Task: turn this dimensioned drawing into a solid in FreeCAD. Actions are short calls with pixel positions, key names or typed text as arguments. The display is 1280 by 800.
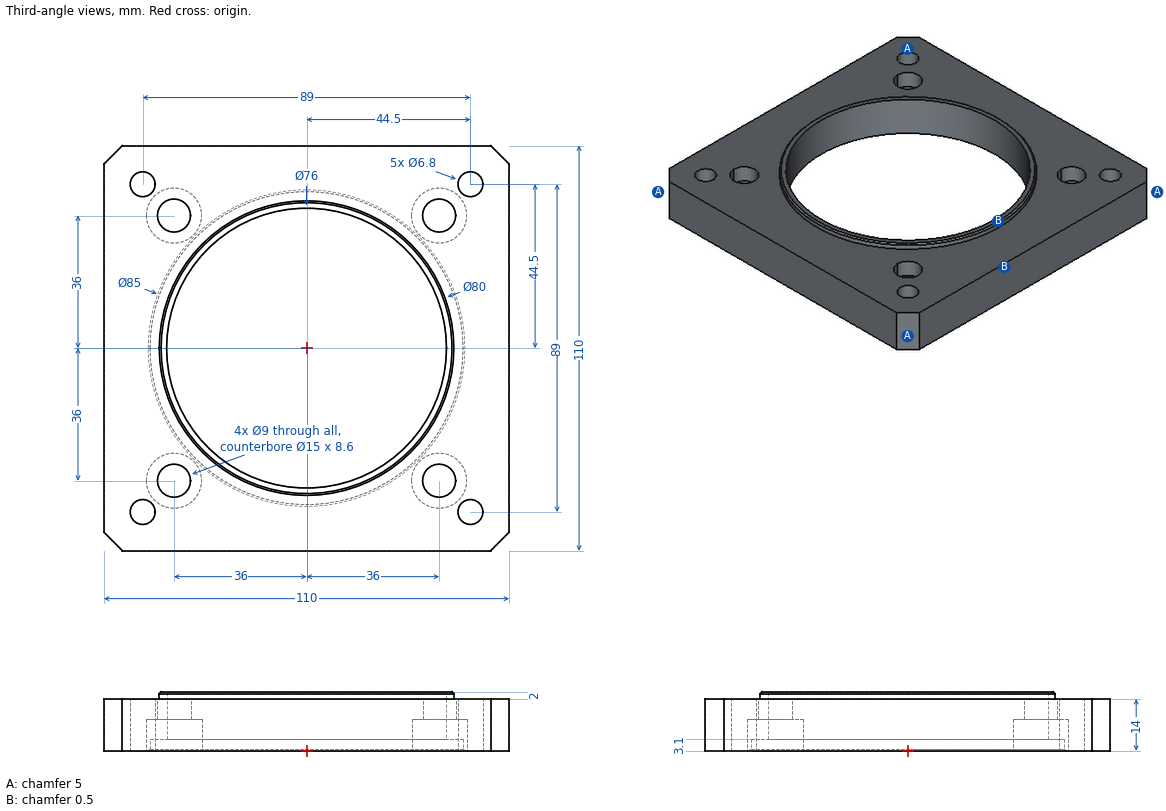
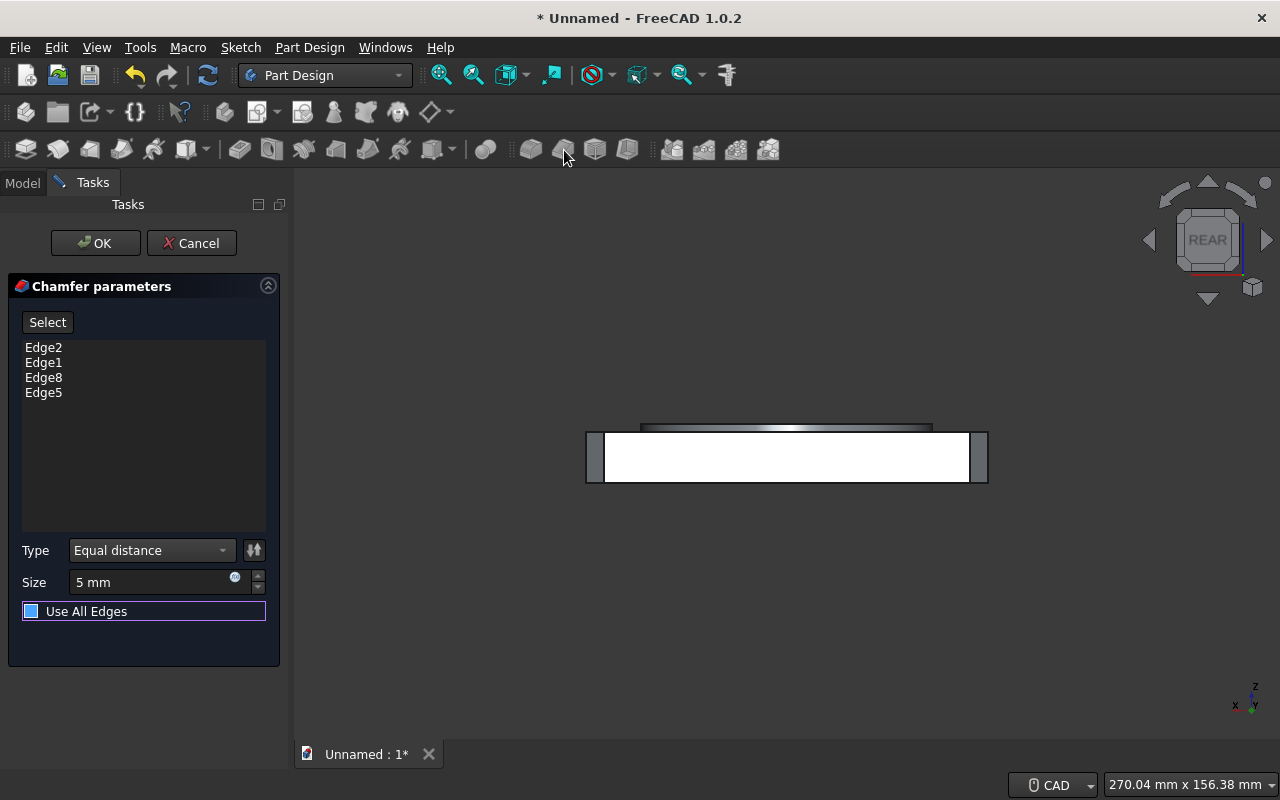
click(96, 243)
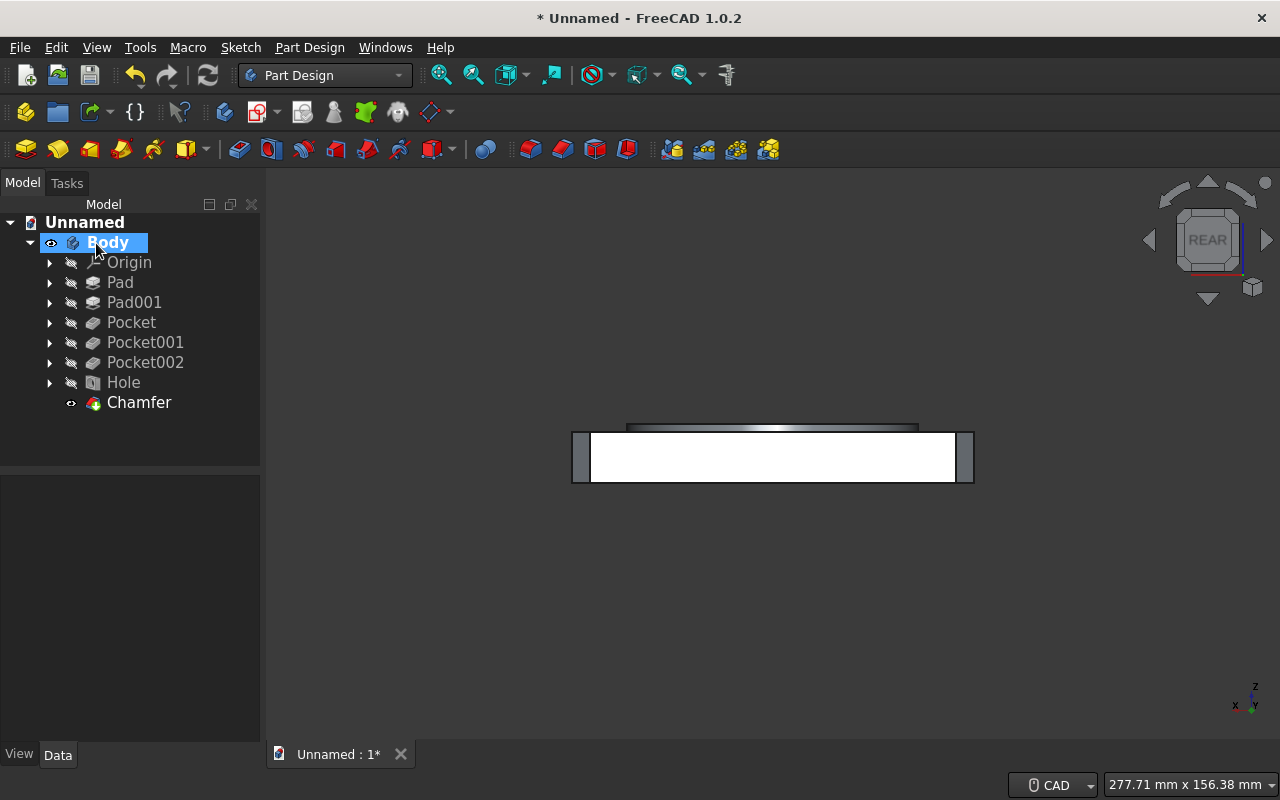
click(442, 76)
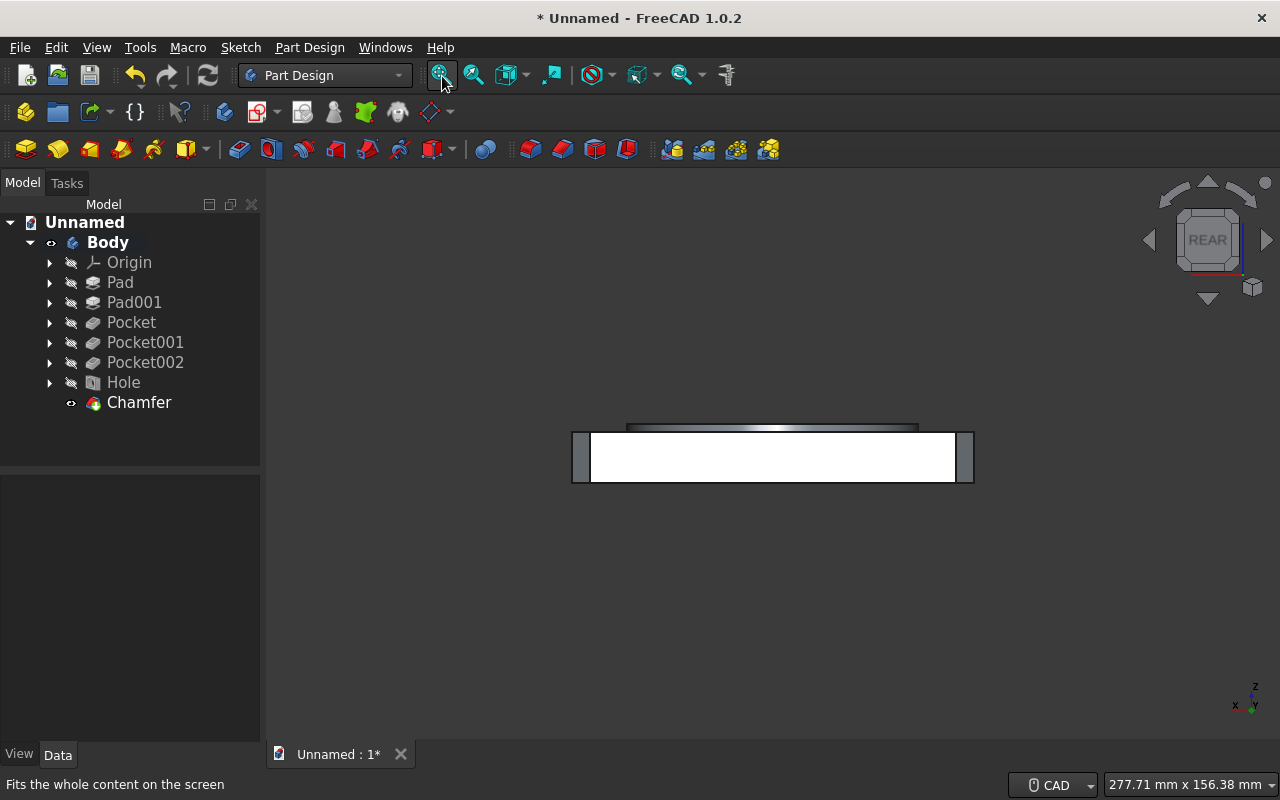
click(891, 423)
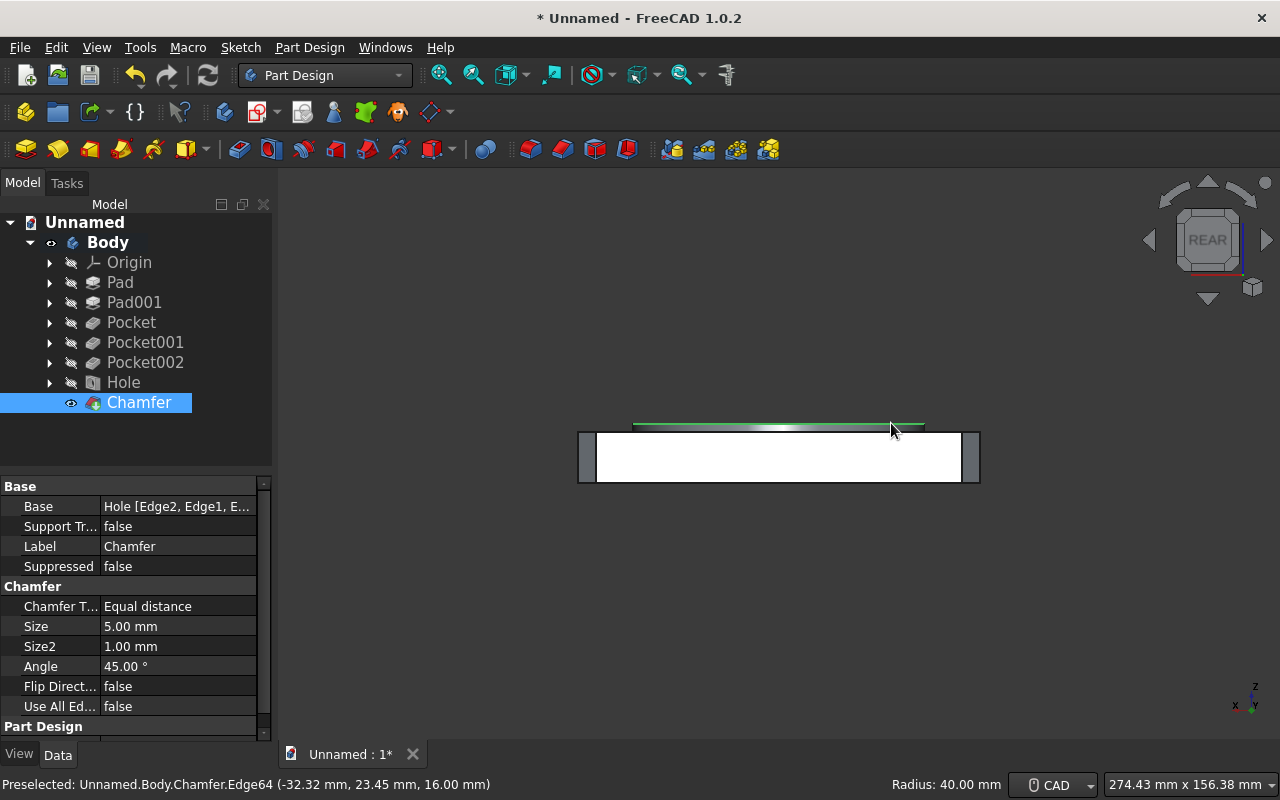
key(0)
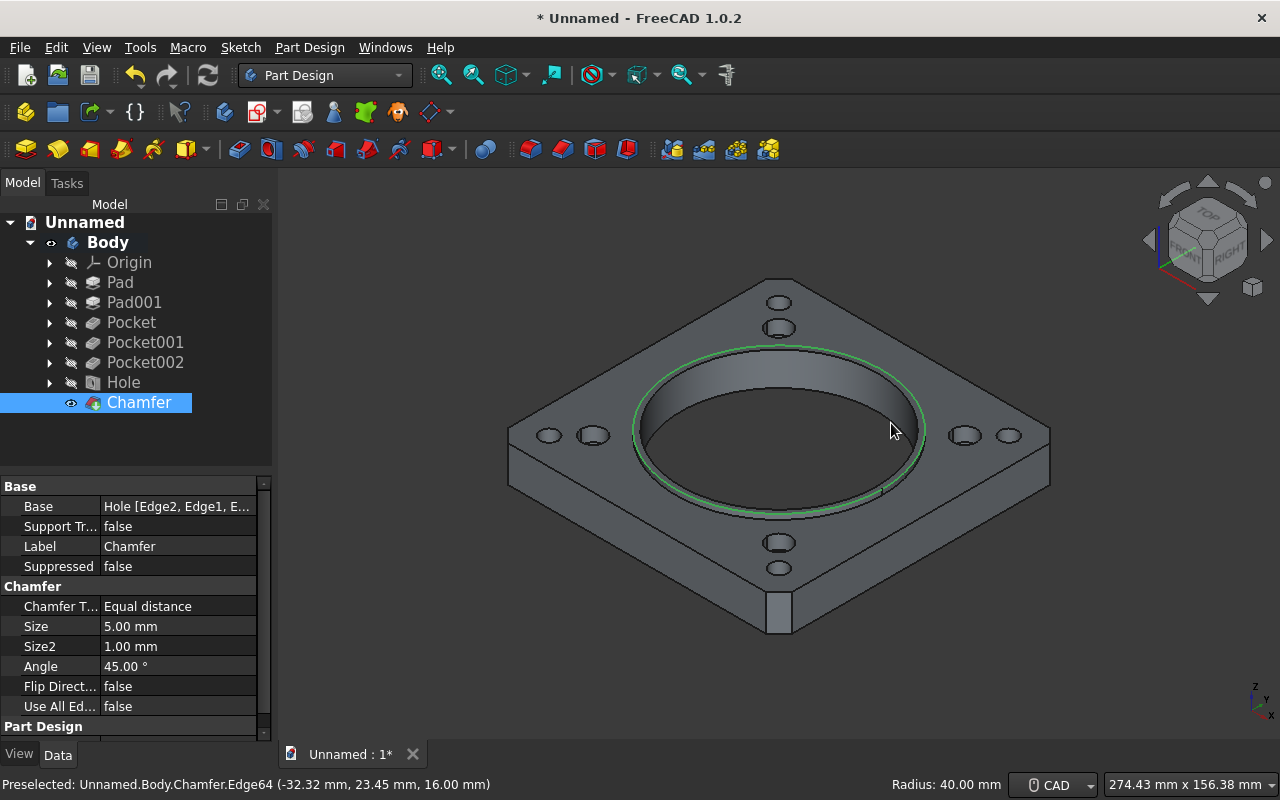
key(2)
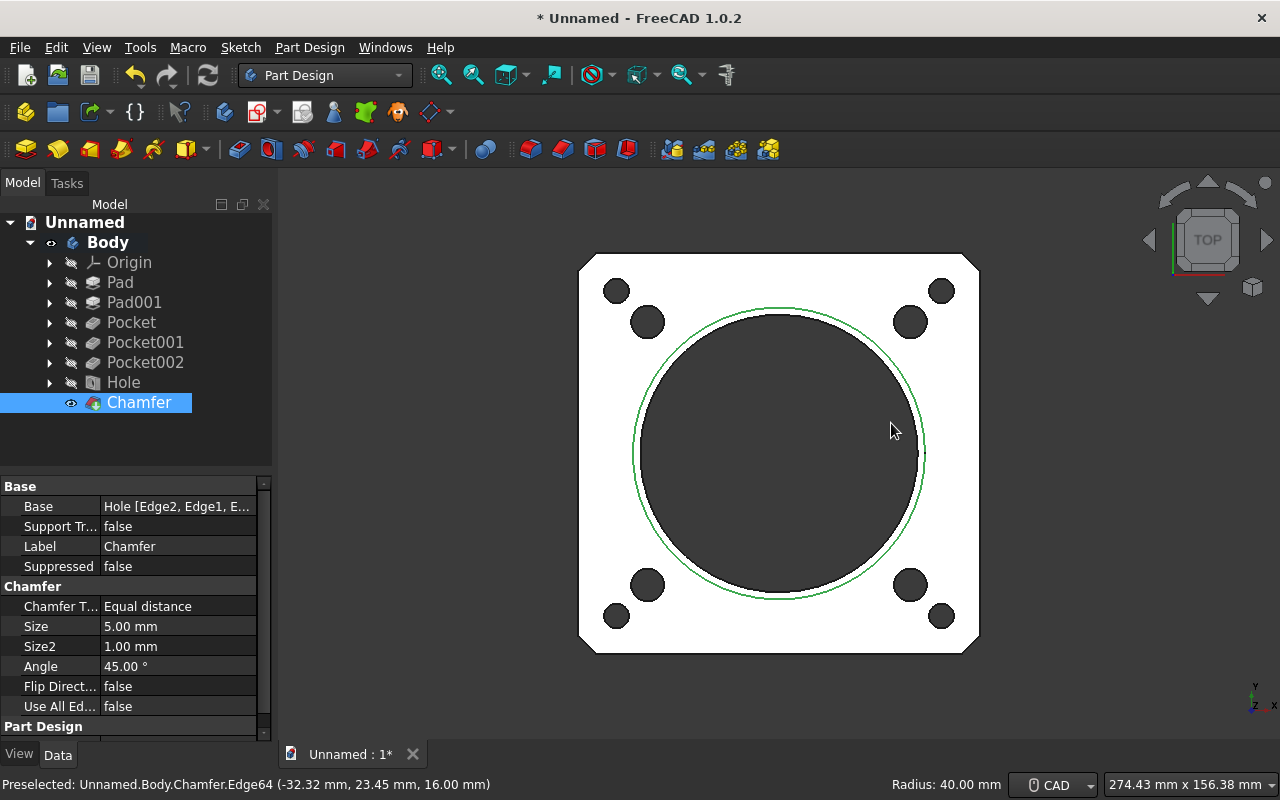
key(1)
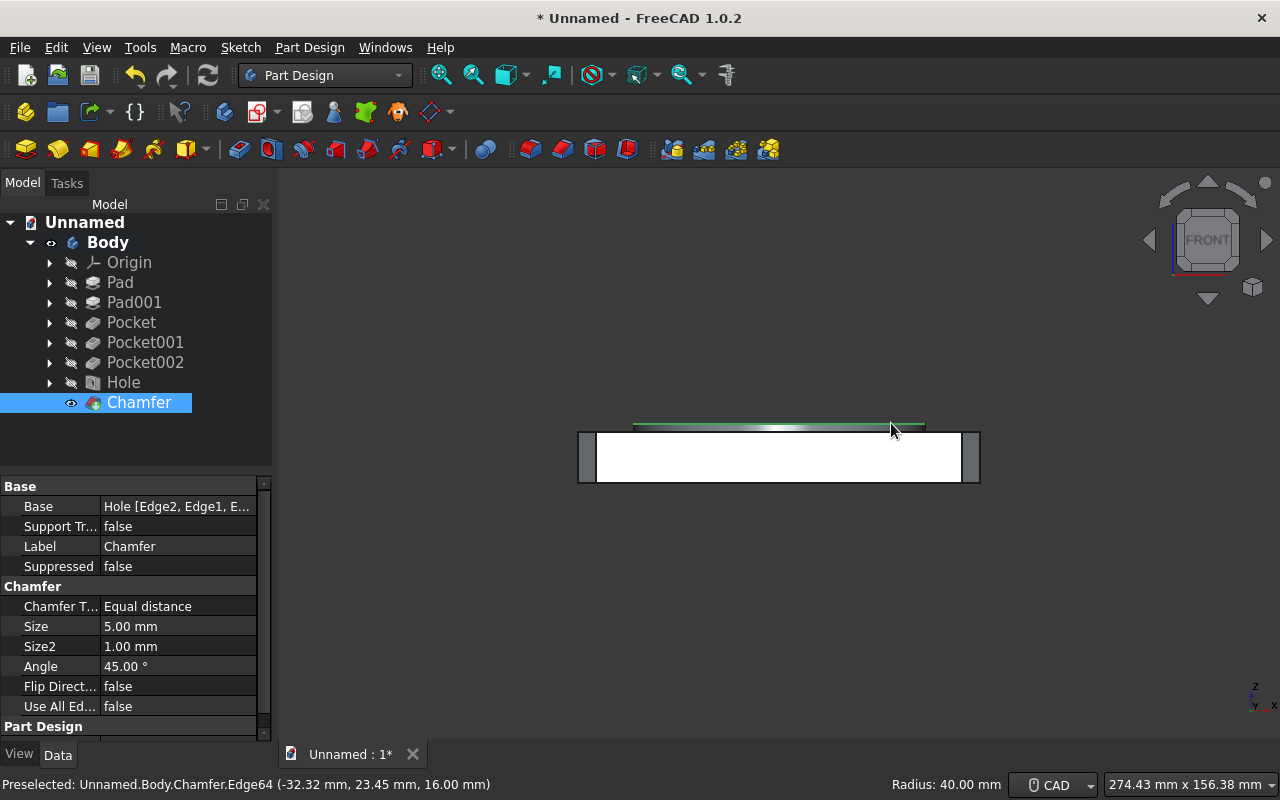
click(442, 76)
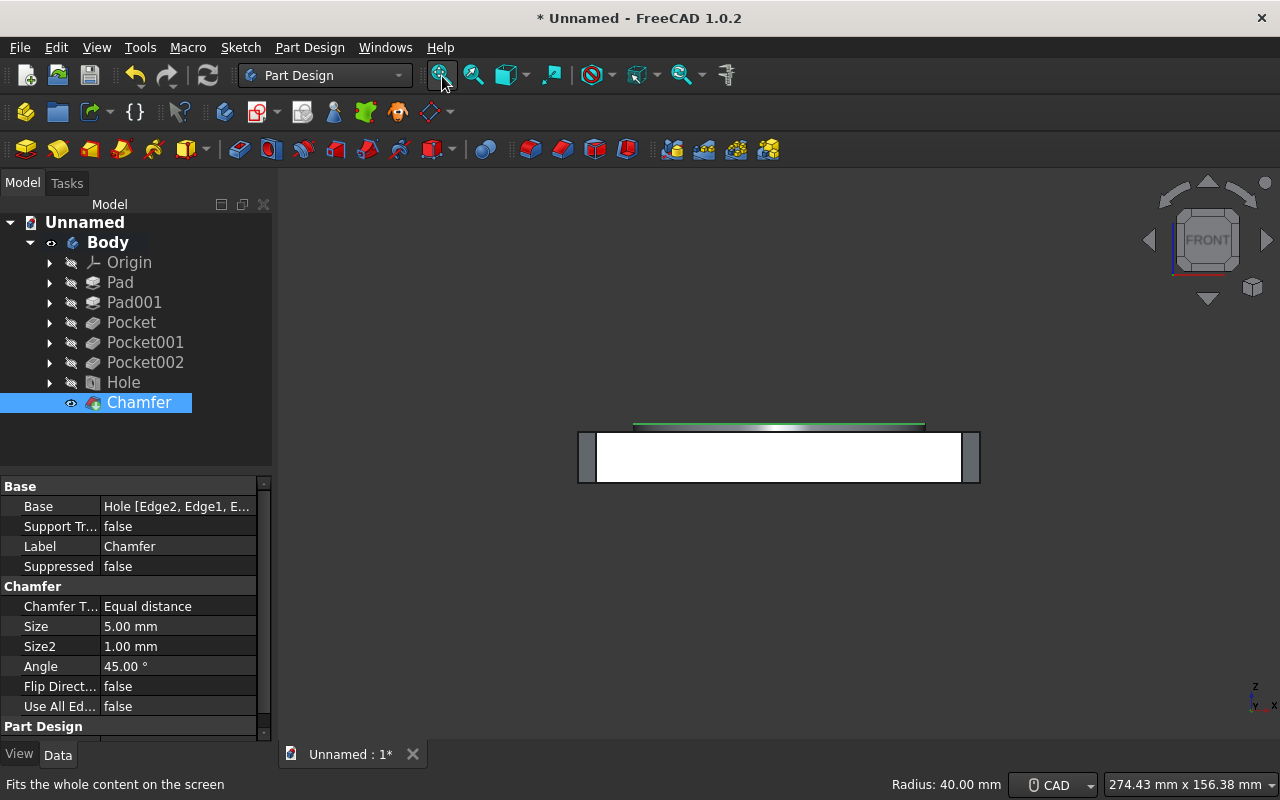
key(3)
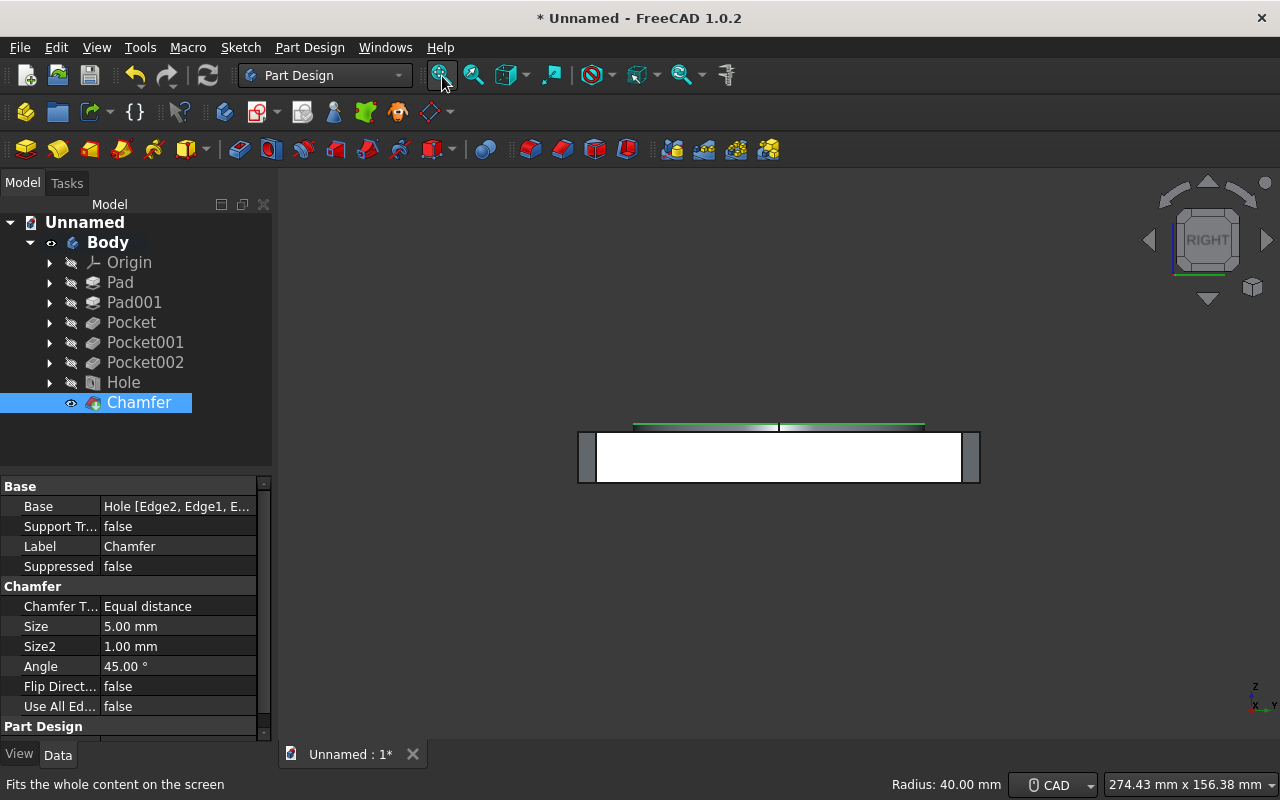
click(442, 76)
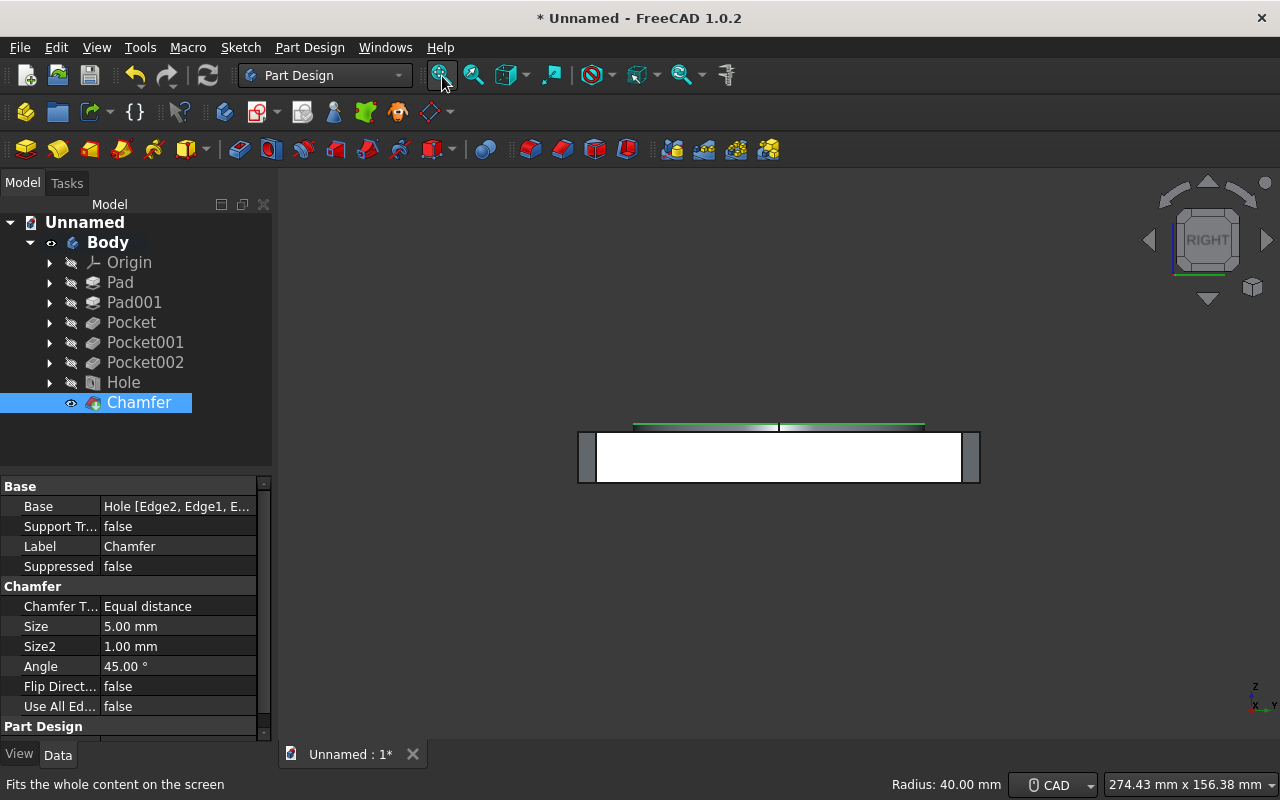
key(5)